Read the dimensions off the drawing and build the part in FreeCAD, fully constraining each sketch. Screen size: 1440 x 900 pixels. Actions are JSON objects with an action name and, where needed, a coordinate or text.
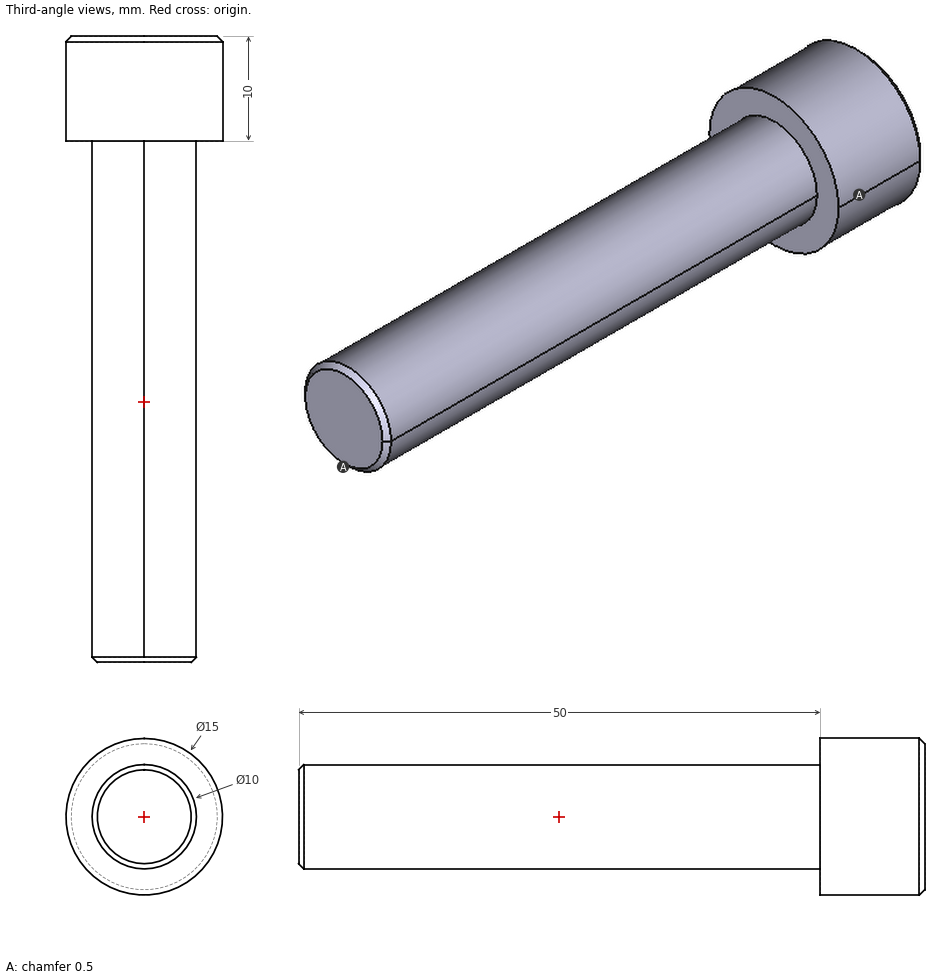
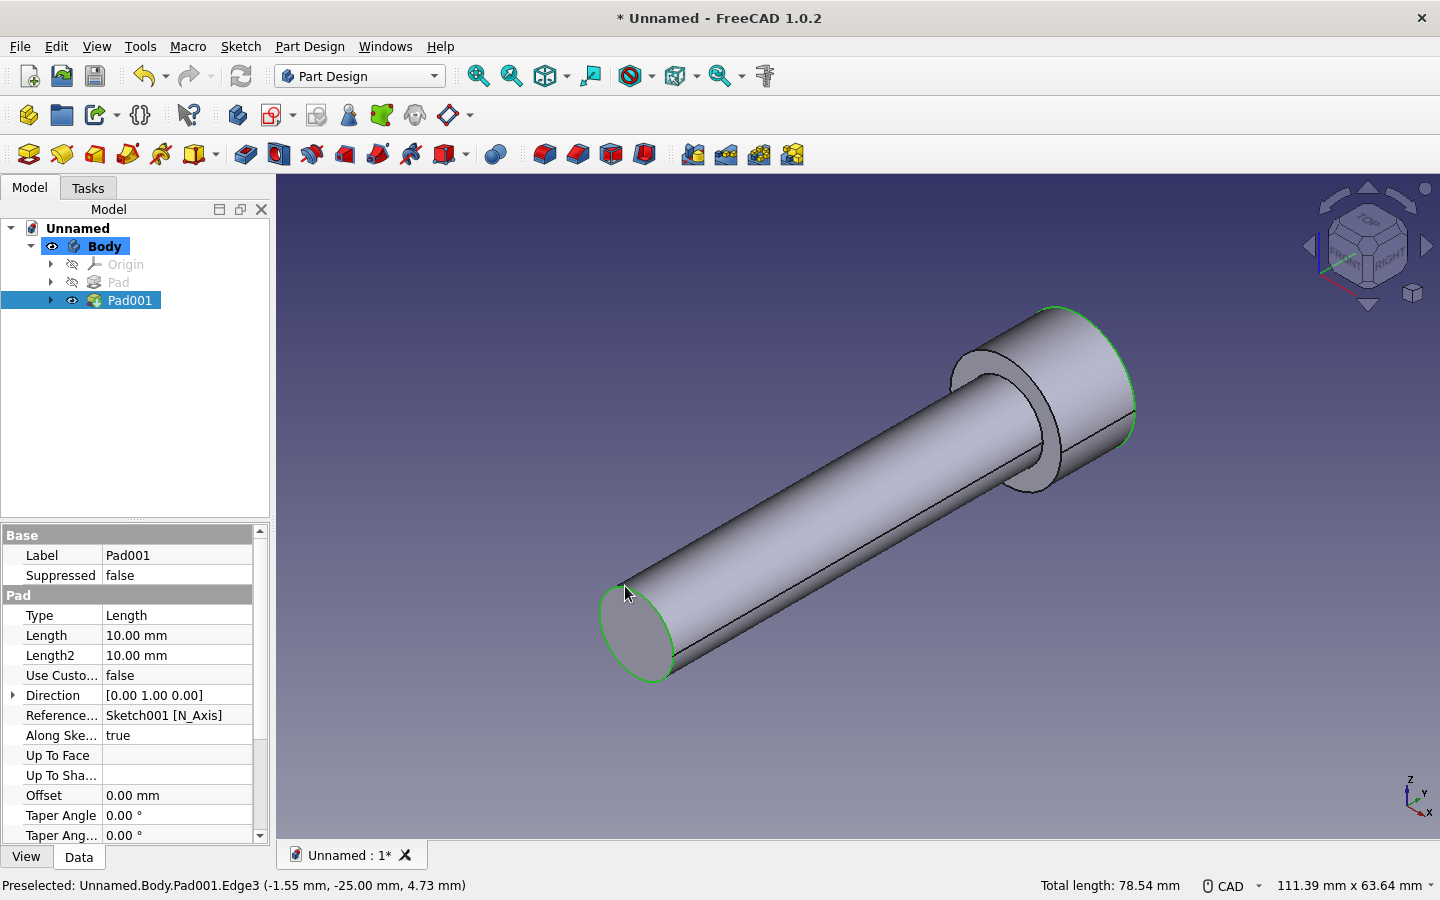
{"action": "left_click", "coordinate": [578, 154]}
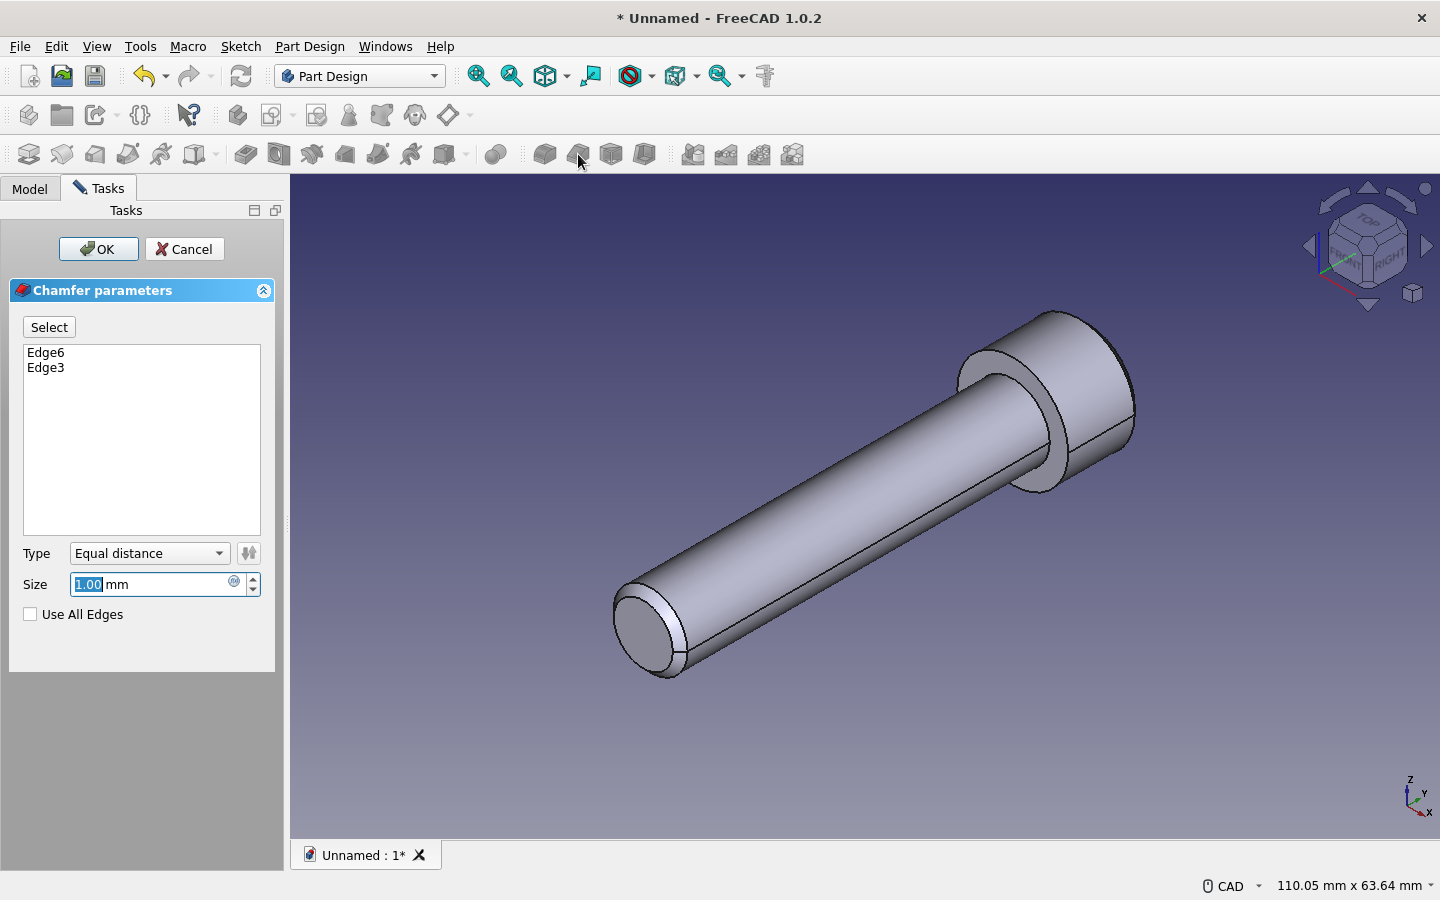
{"action": "type", "text": "0.5"}
{"action": "key", "text": "Tab"}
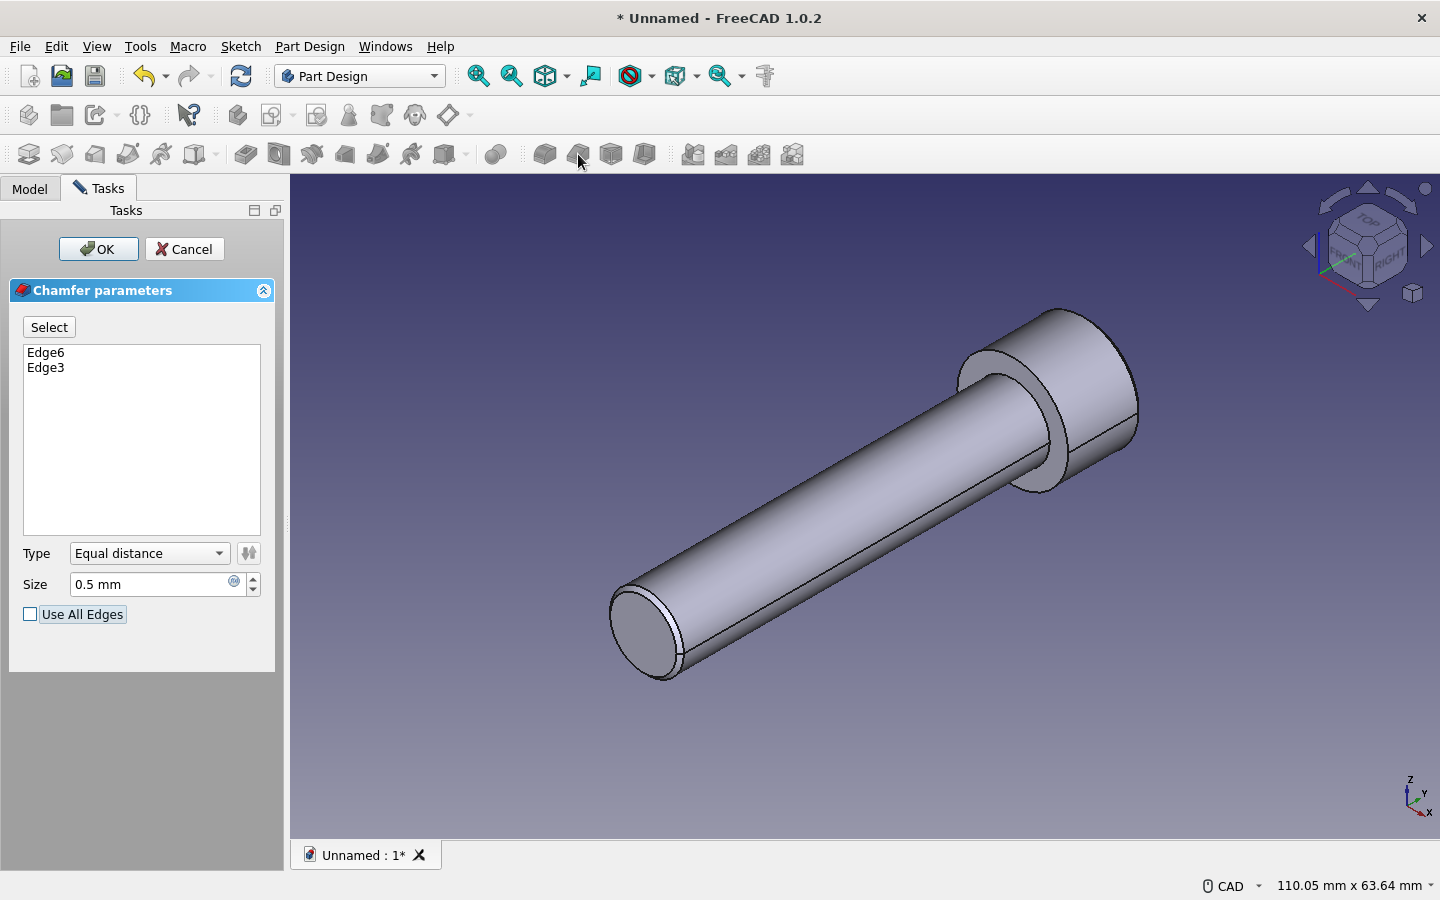
{"action": "left_click", "coordinate": [99, 249]}